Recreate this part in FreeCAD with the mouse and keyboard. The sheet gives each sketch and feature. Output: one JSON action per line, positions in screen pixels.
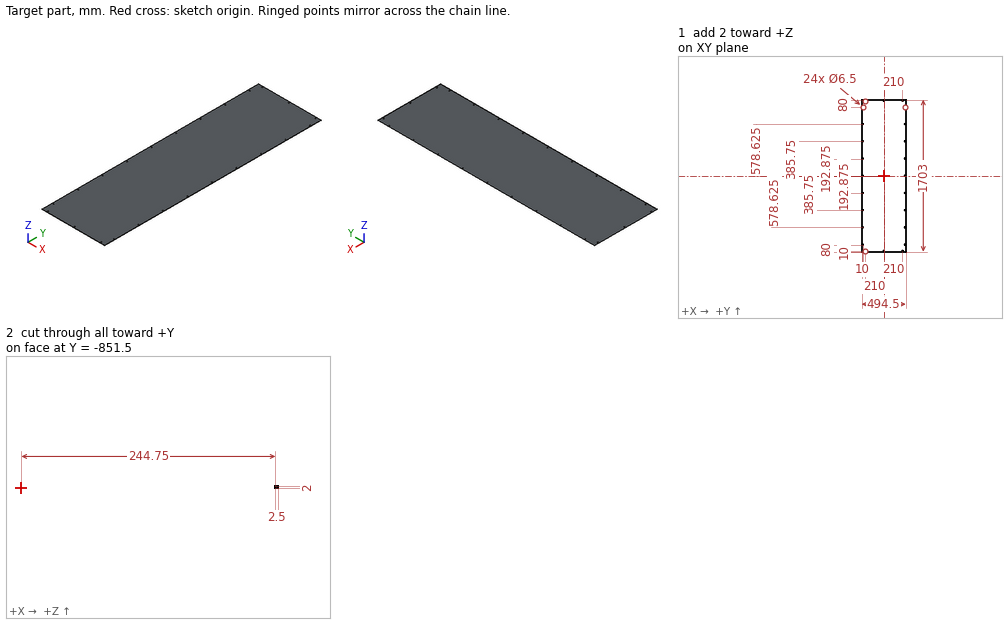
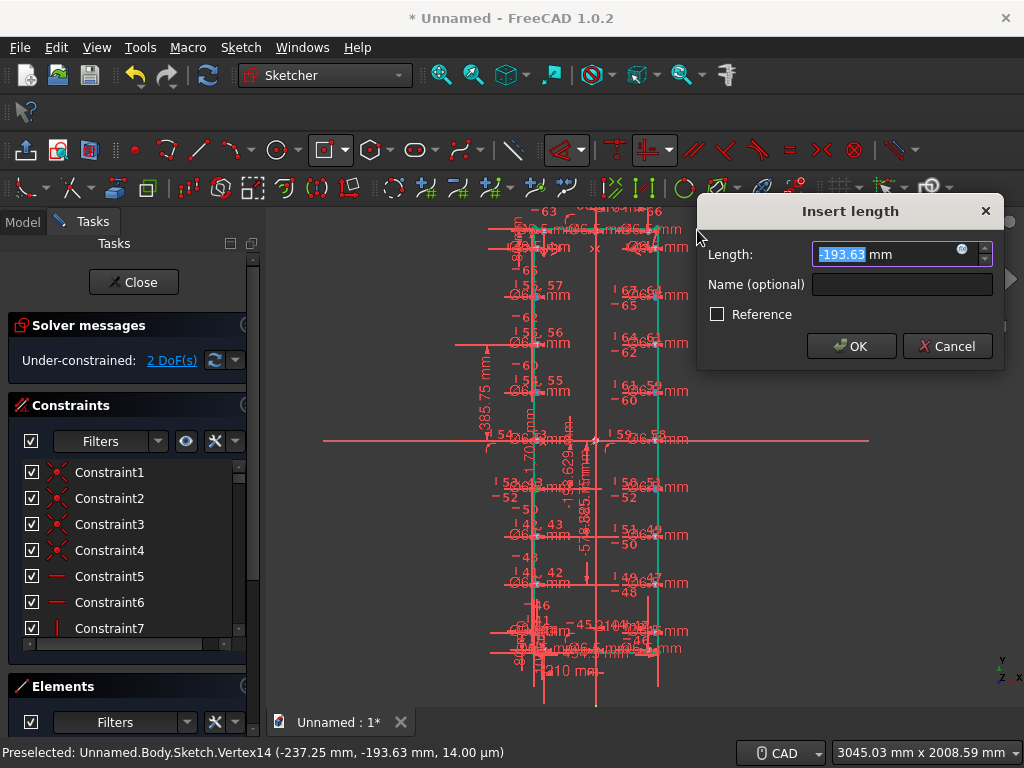
{"action": "type", "text": "-192.875"}
{"action": "key", "text": "Return"}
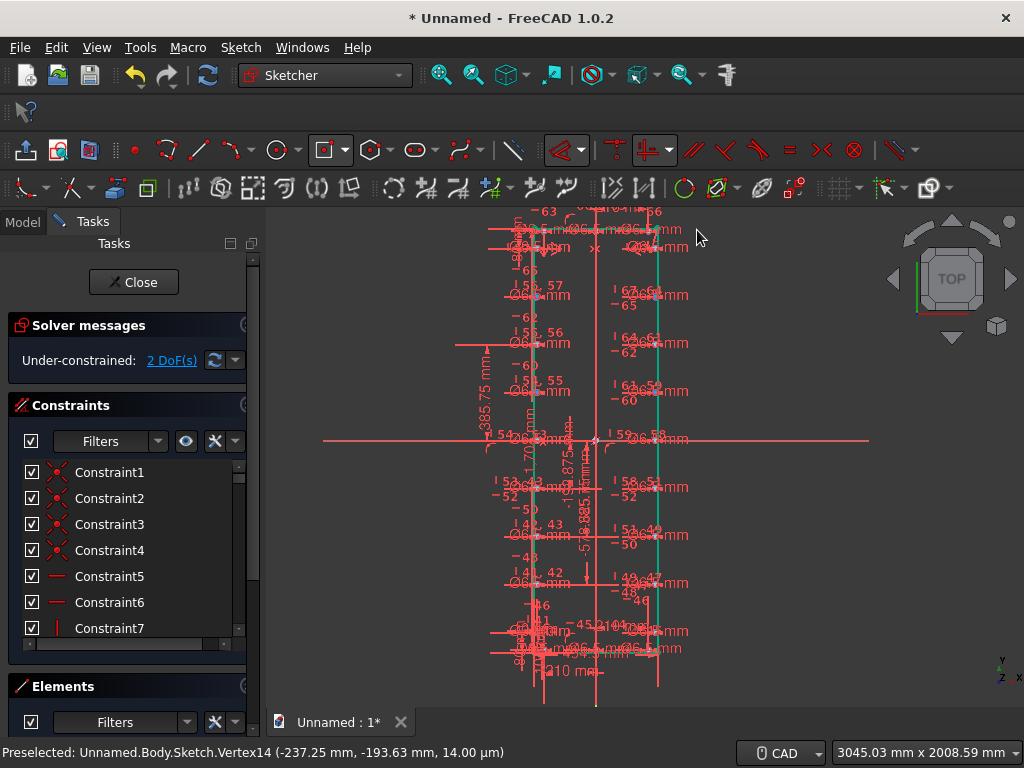
{"action": "left_click", "coordinate": [537, 393]}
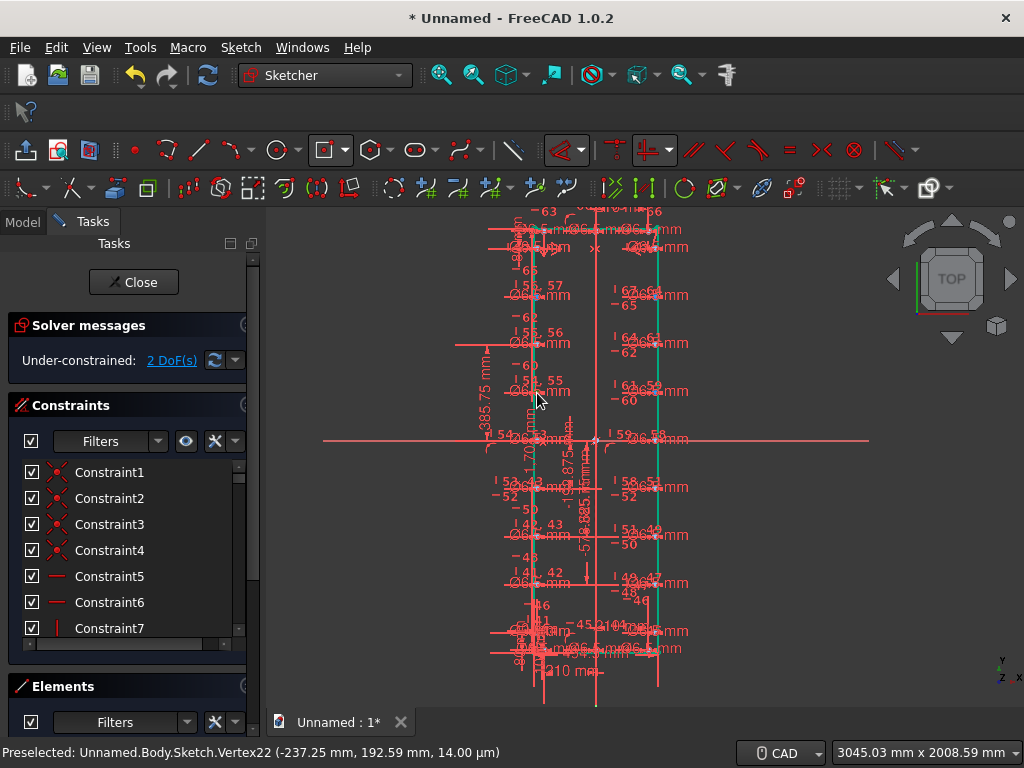
{"action": "left_click", "coordinate": [584, 150]}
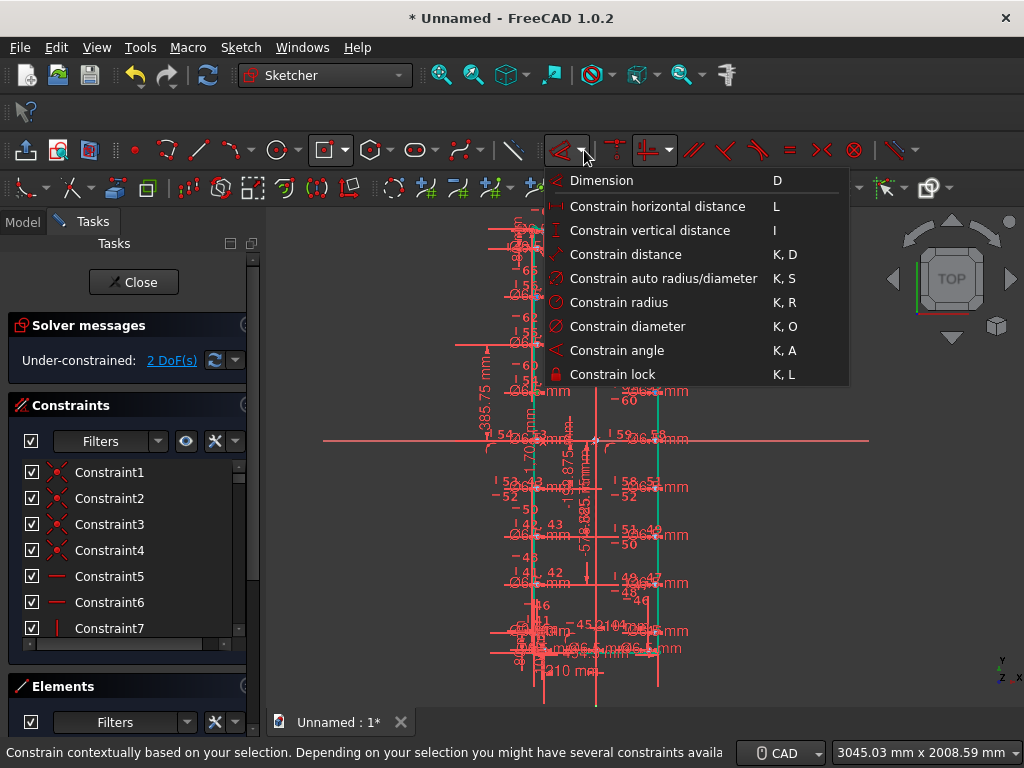
{"action": "left_click", "coordinate": [697, 230]}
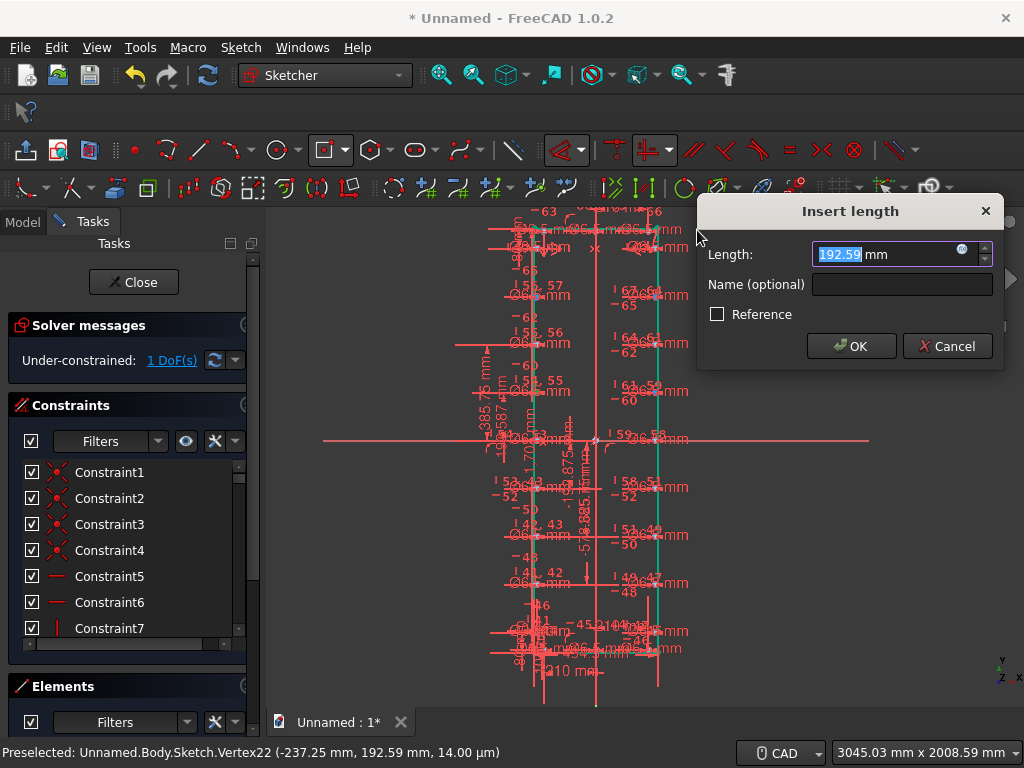
{"action": "type", "text": "192.875"}
{"action": "key", "text": "Return"}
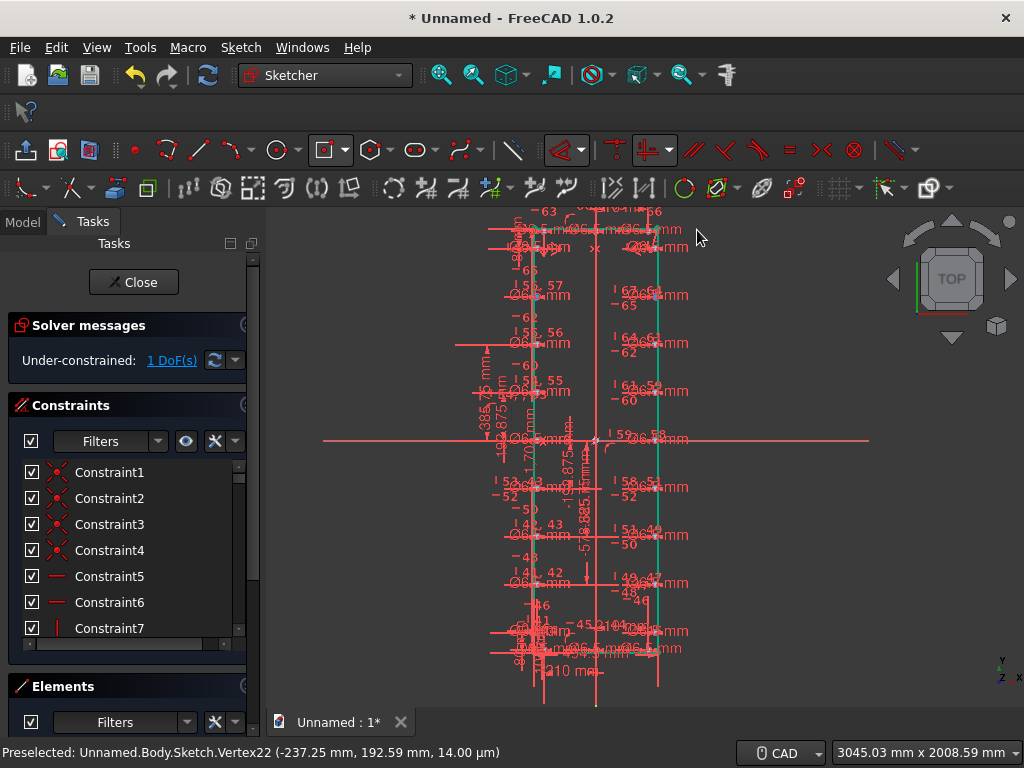
{"action": "left_click", "coordinate": [537, 297]}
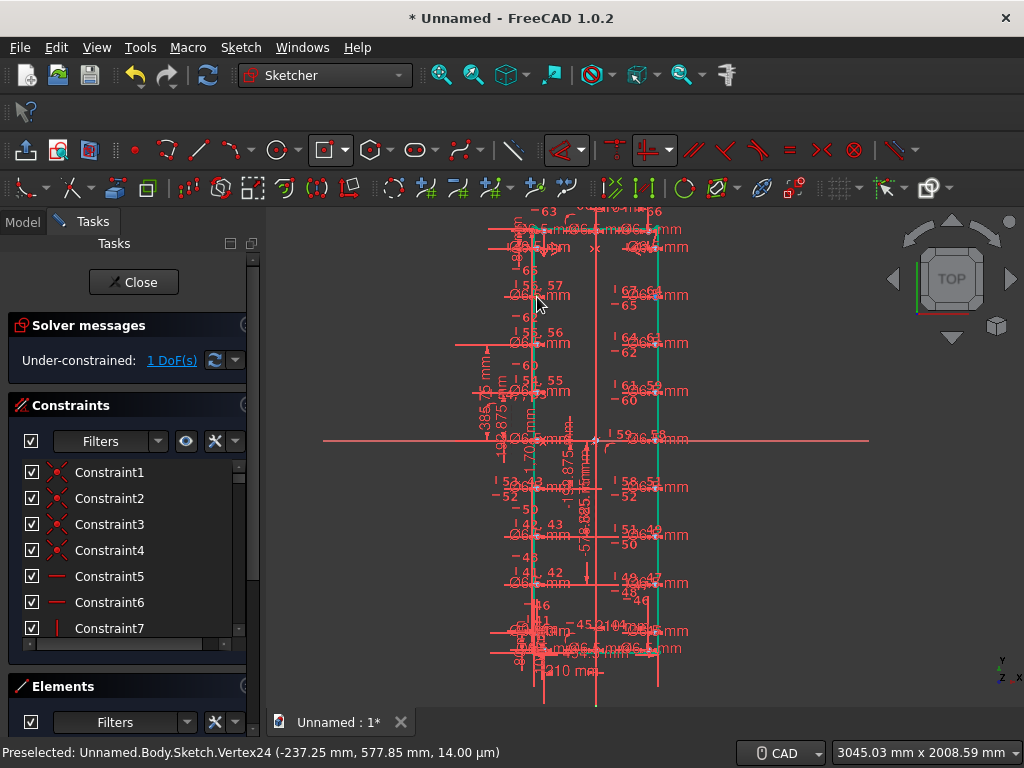
{"action": "left_click", "coordinate": [584, 150]}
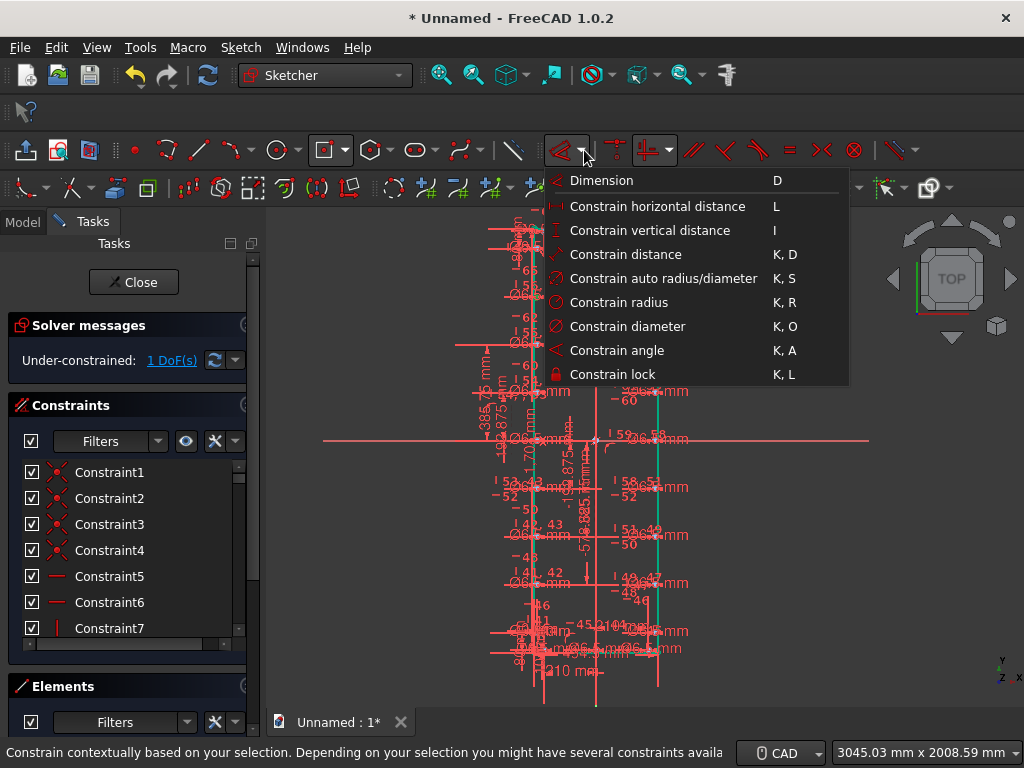
{"action": "left_click", "coordinate": [697, 230]}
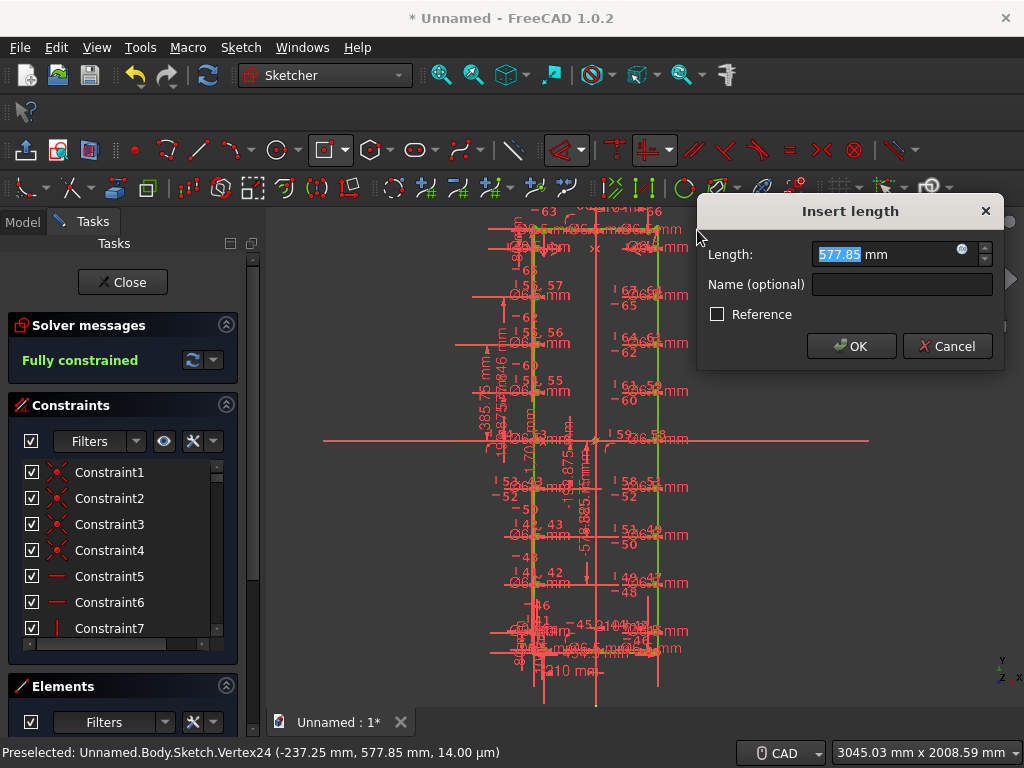
{"action": "type", "text": "578.625"}
{"action": "key", "text": "Return"}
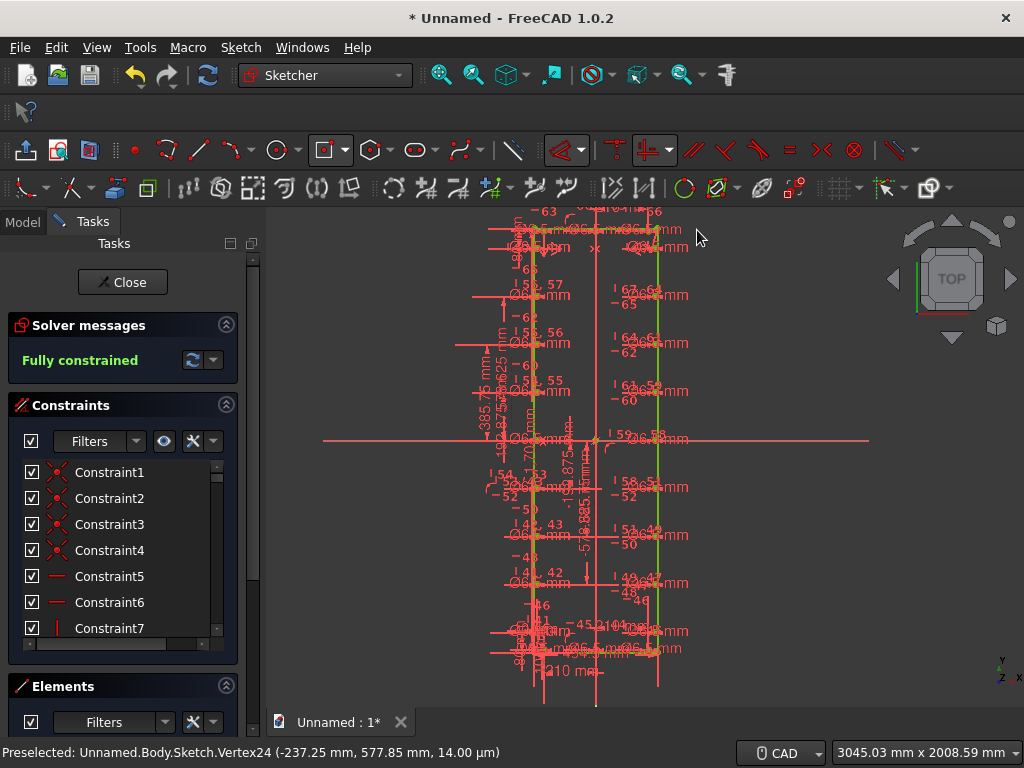
{"action": "left_click", "coordinate": [123, 282]}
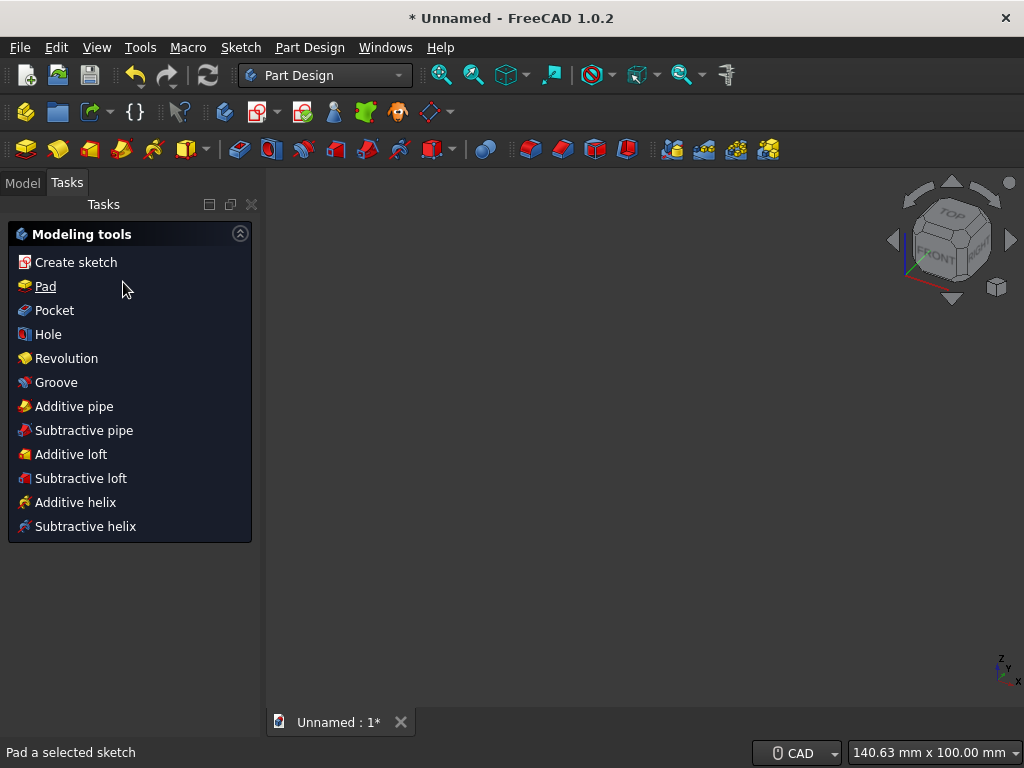
{"action": "left_click", "coordinate": [26, 150]}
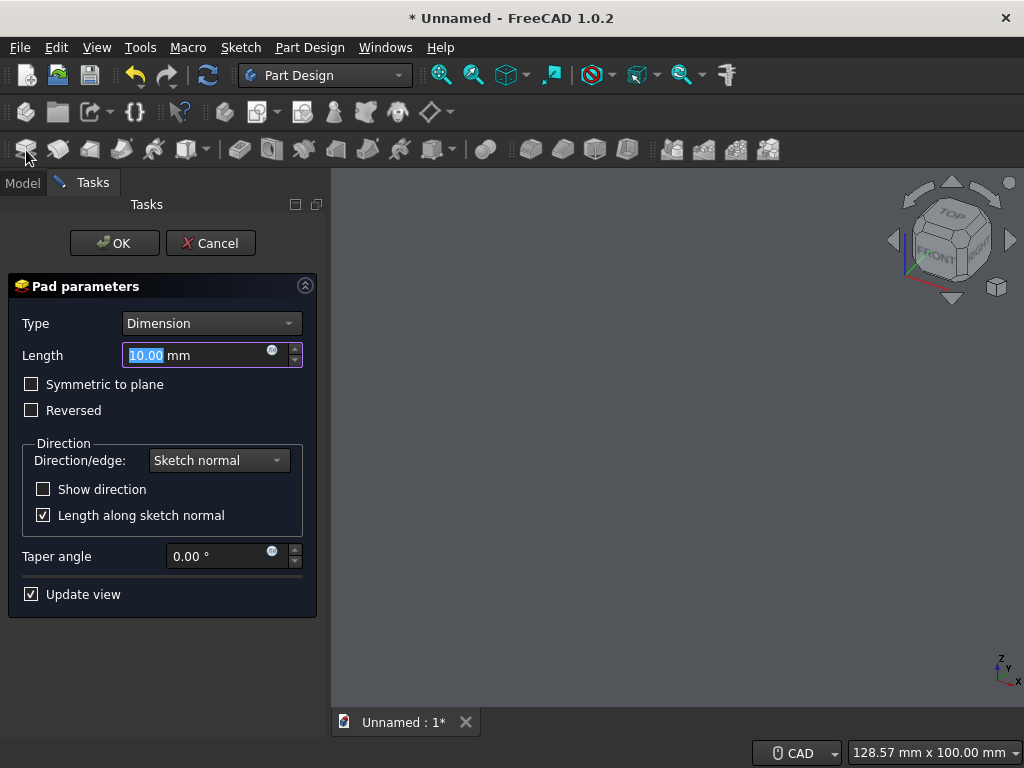
{"action": "type", "text": "2"}
{"action": "key", "text": "Tab"}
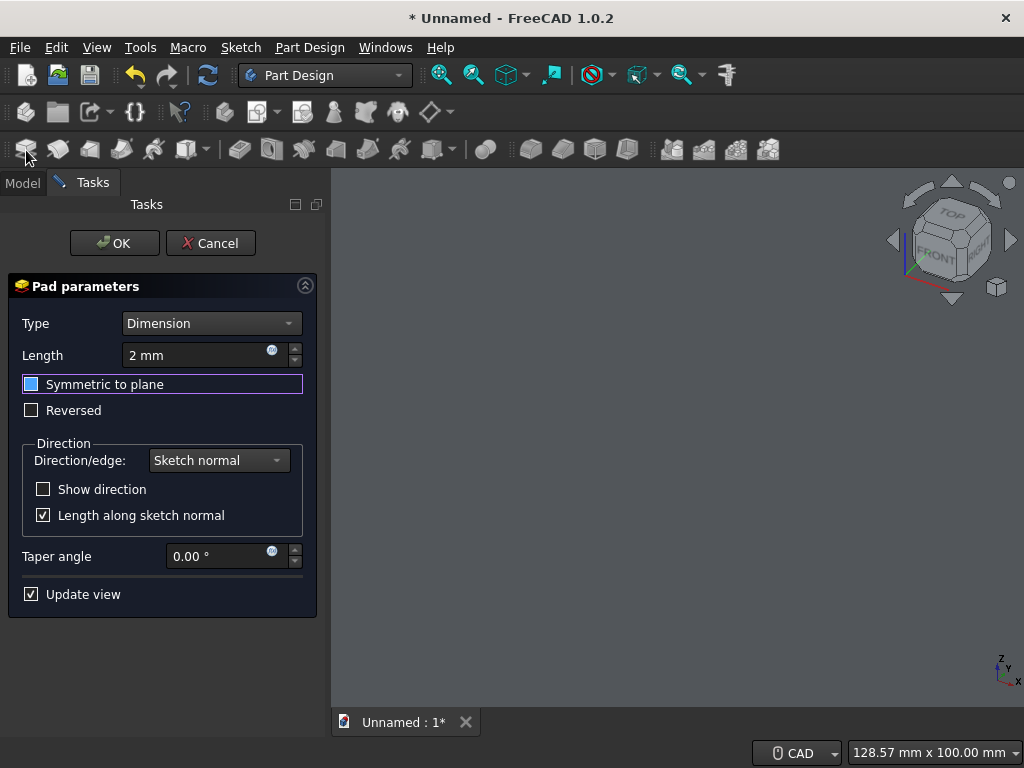
{"action": "left_click", "coordinate": [115, 243]}